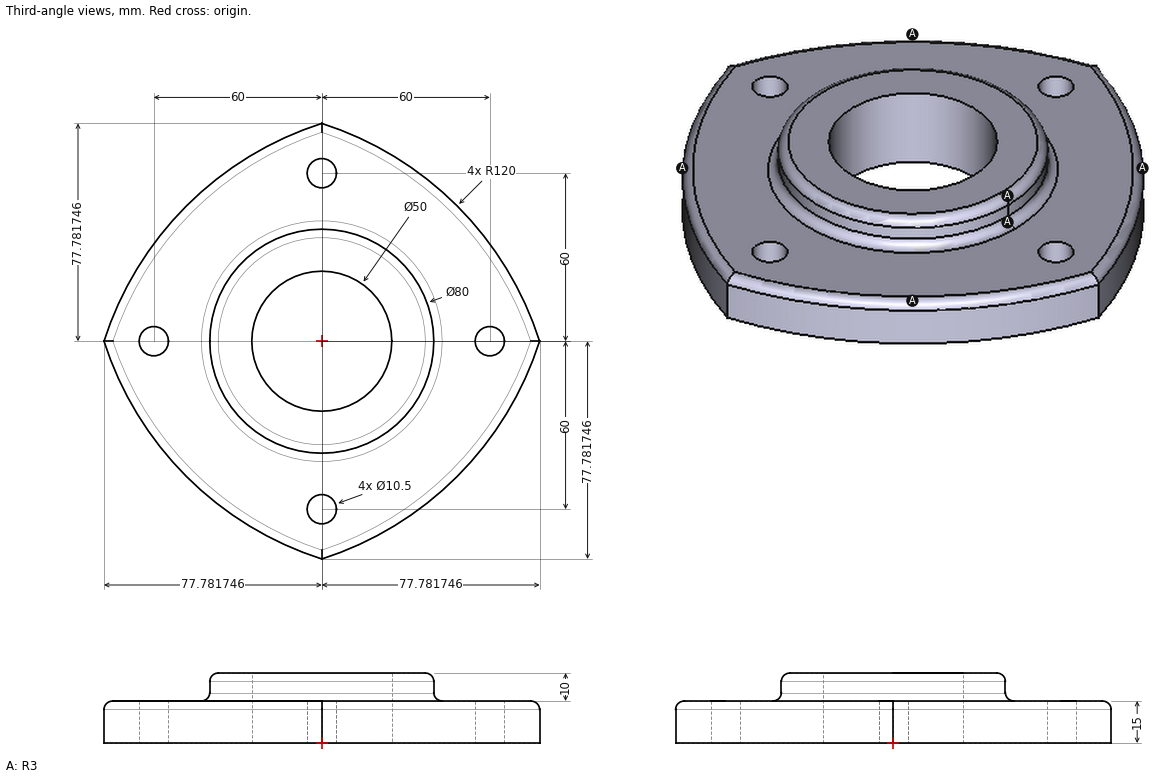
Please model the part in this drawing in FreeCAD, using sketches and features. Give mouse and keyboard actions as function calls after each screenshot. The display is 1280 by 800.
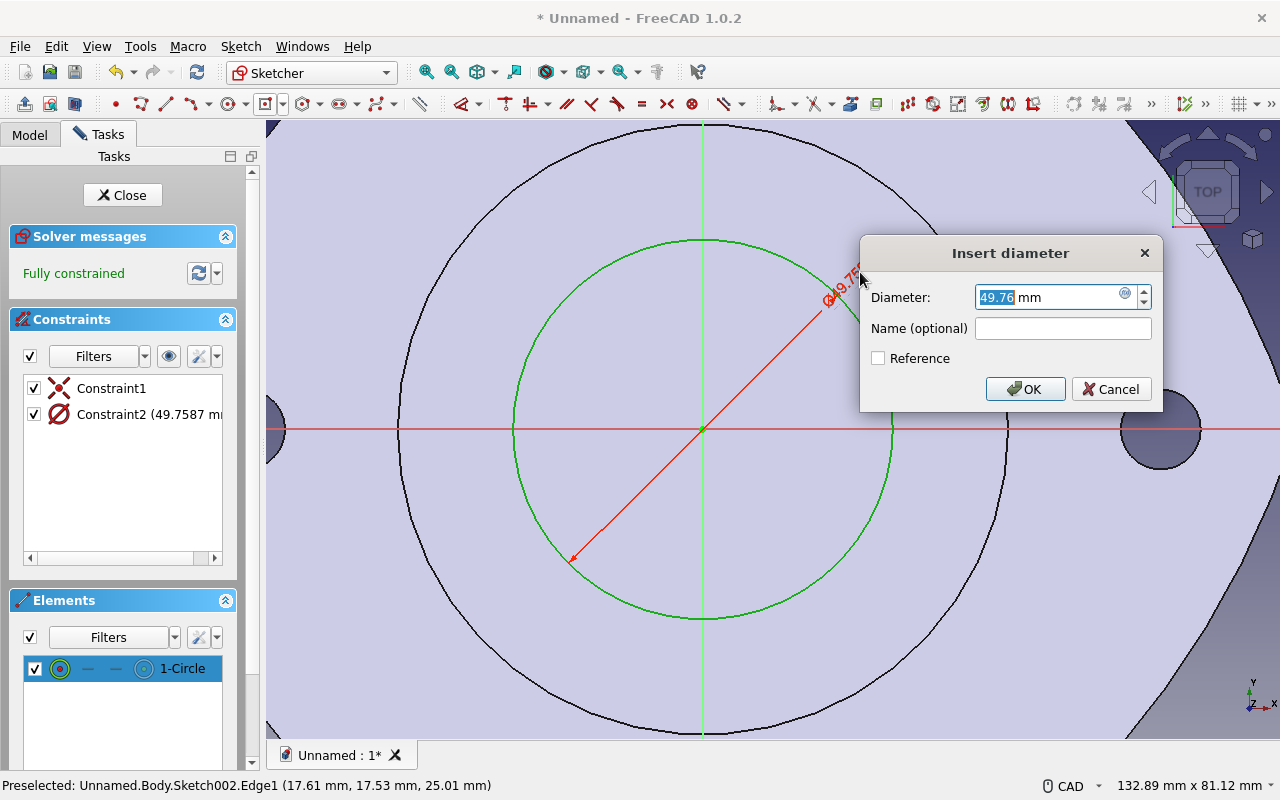
text(50)
key(Return)
key(Escape)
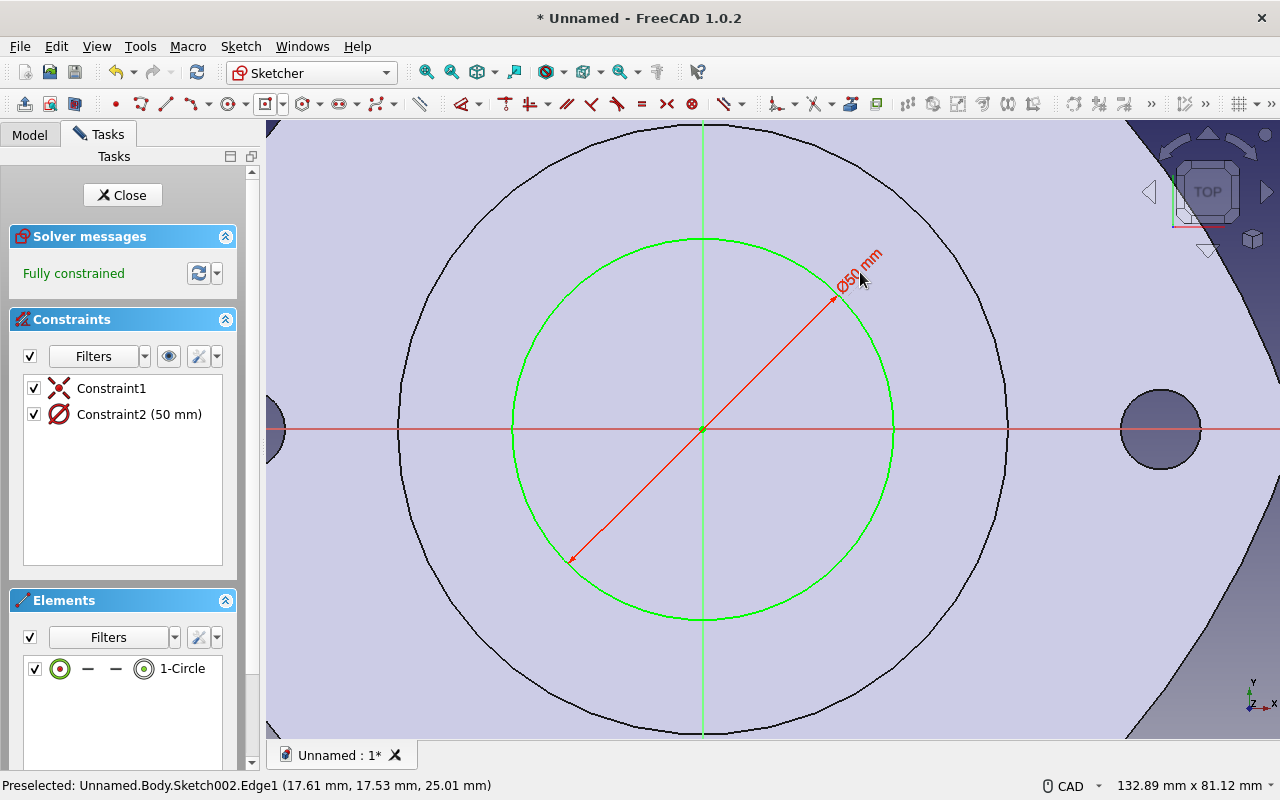
click(123, 195)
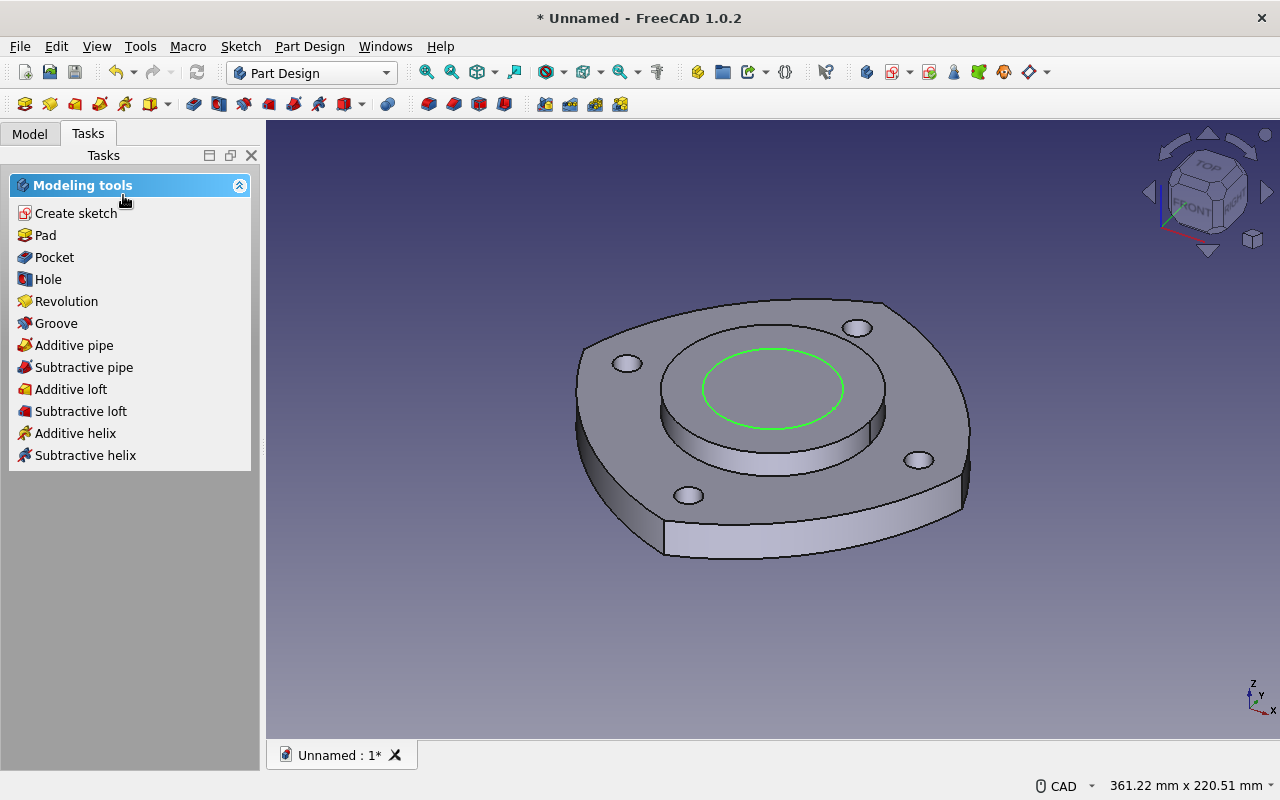
click(194, 104)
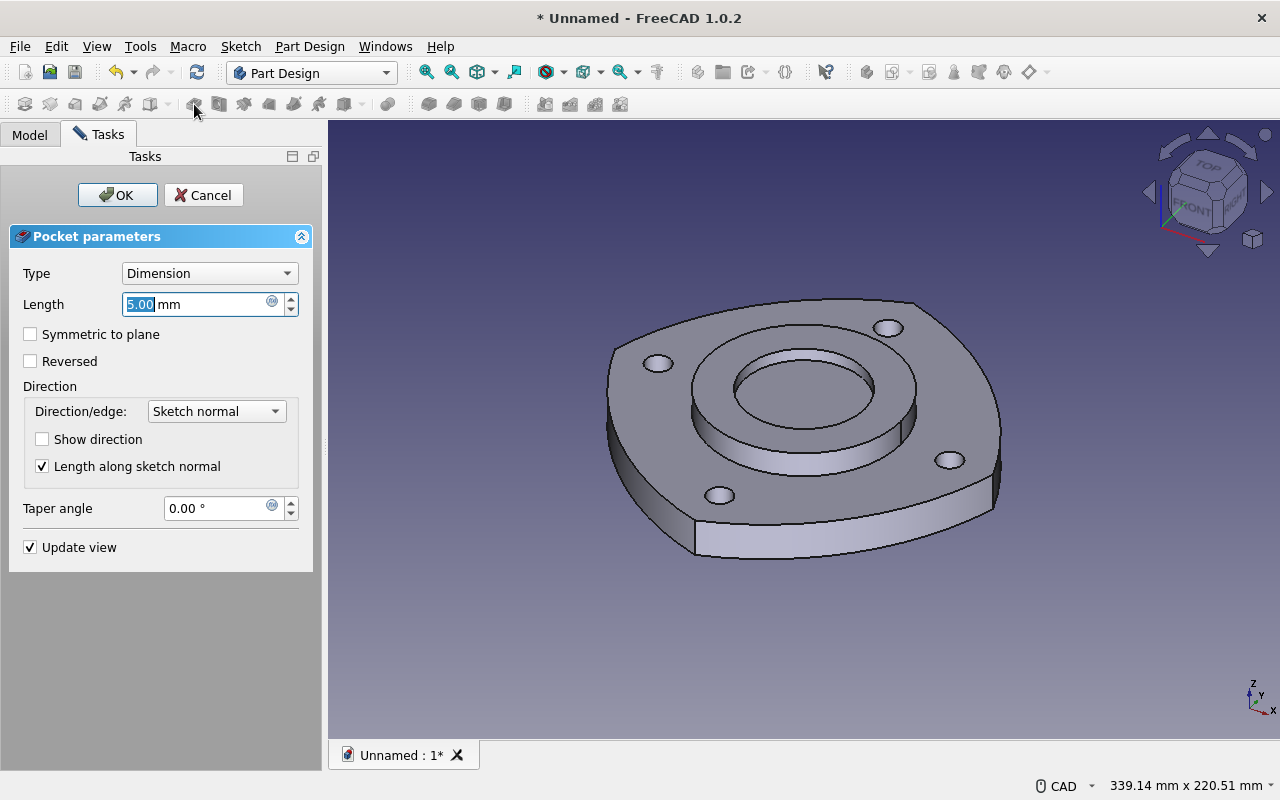
click(210, 274)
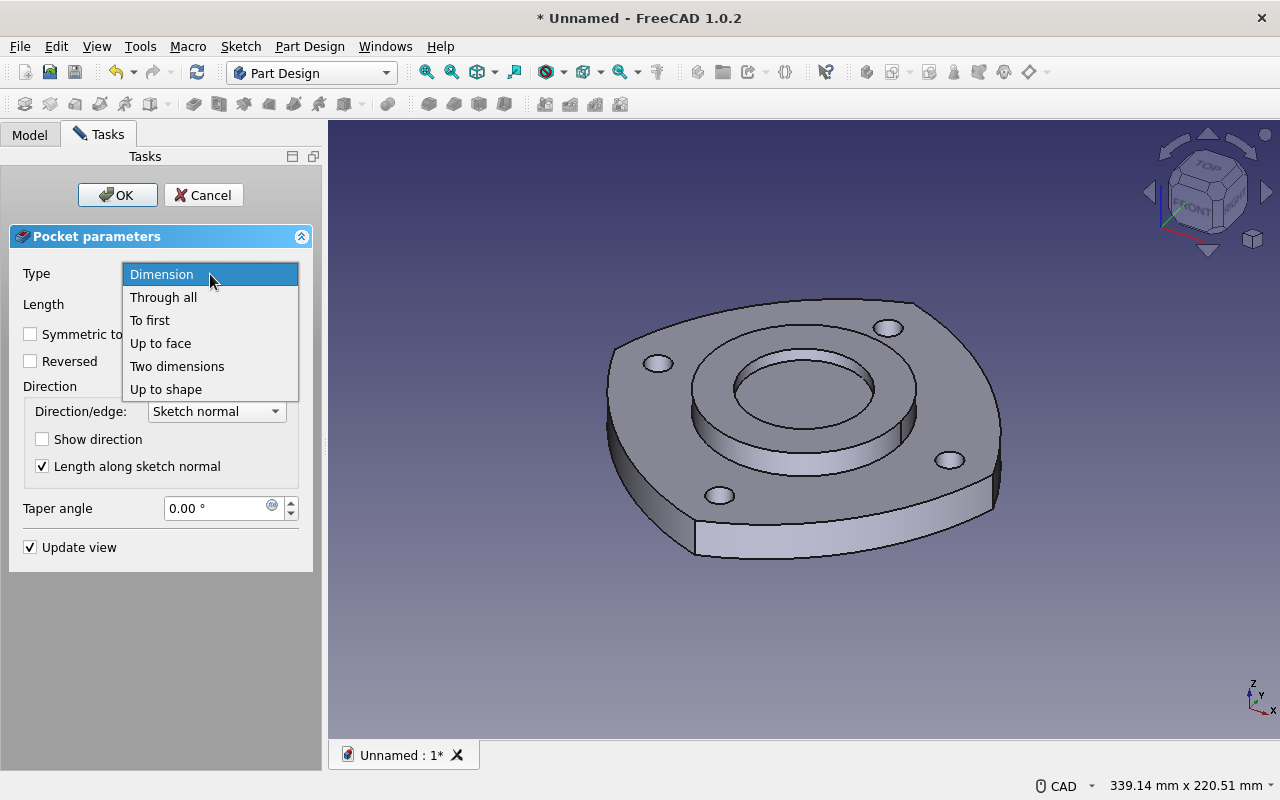
click(208, 298)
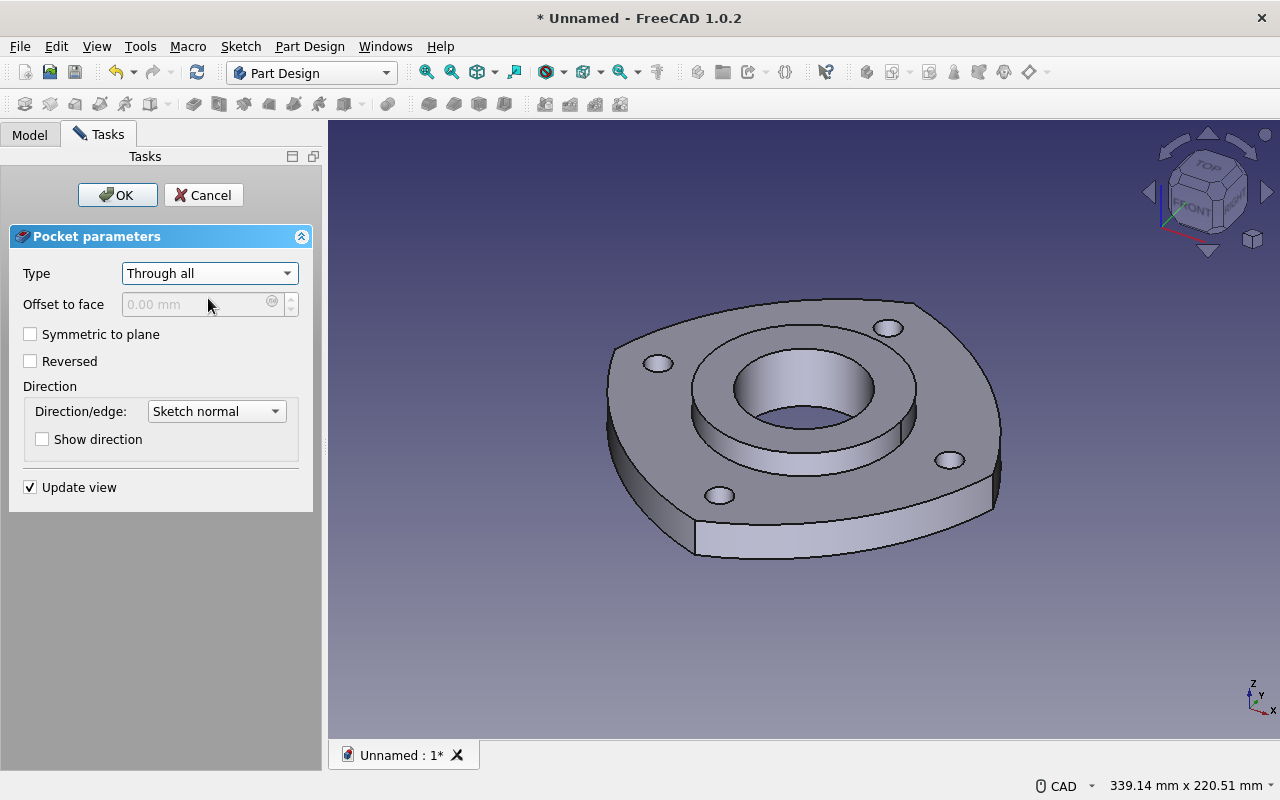
click(118, 195)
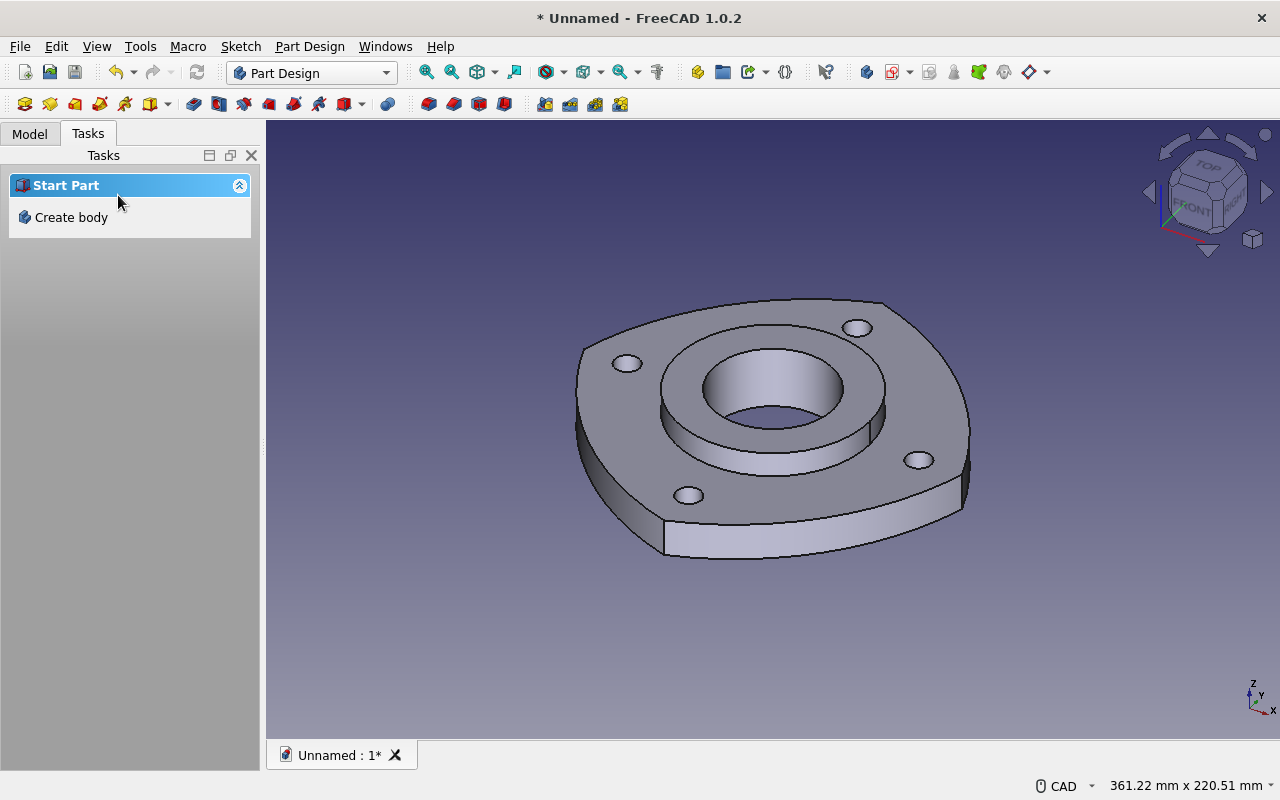
click(823, 517)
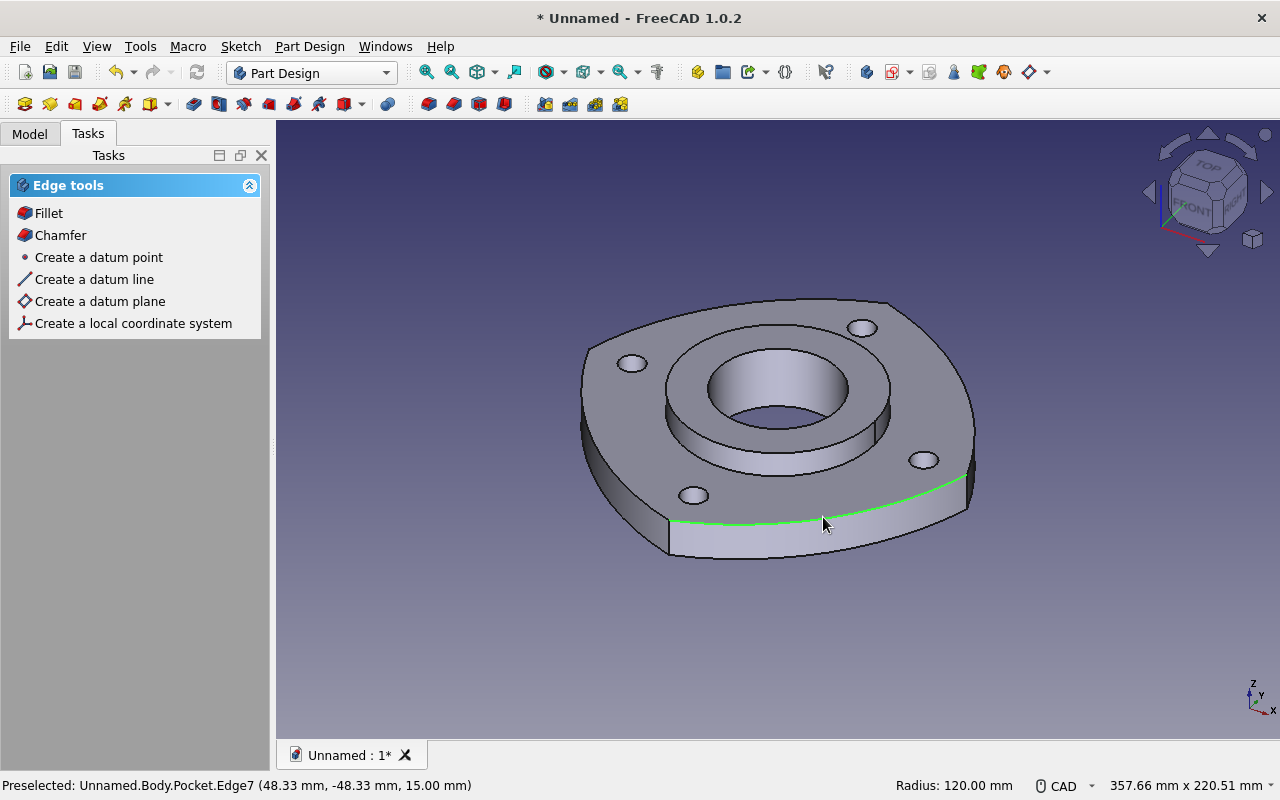
click(954, 365, ctrl)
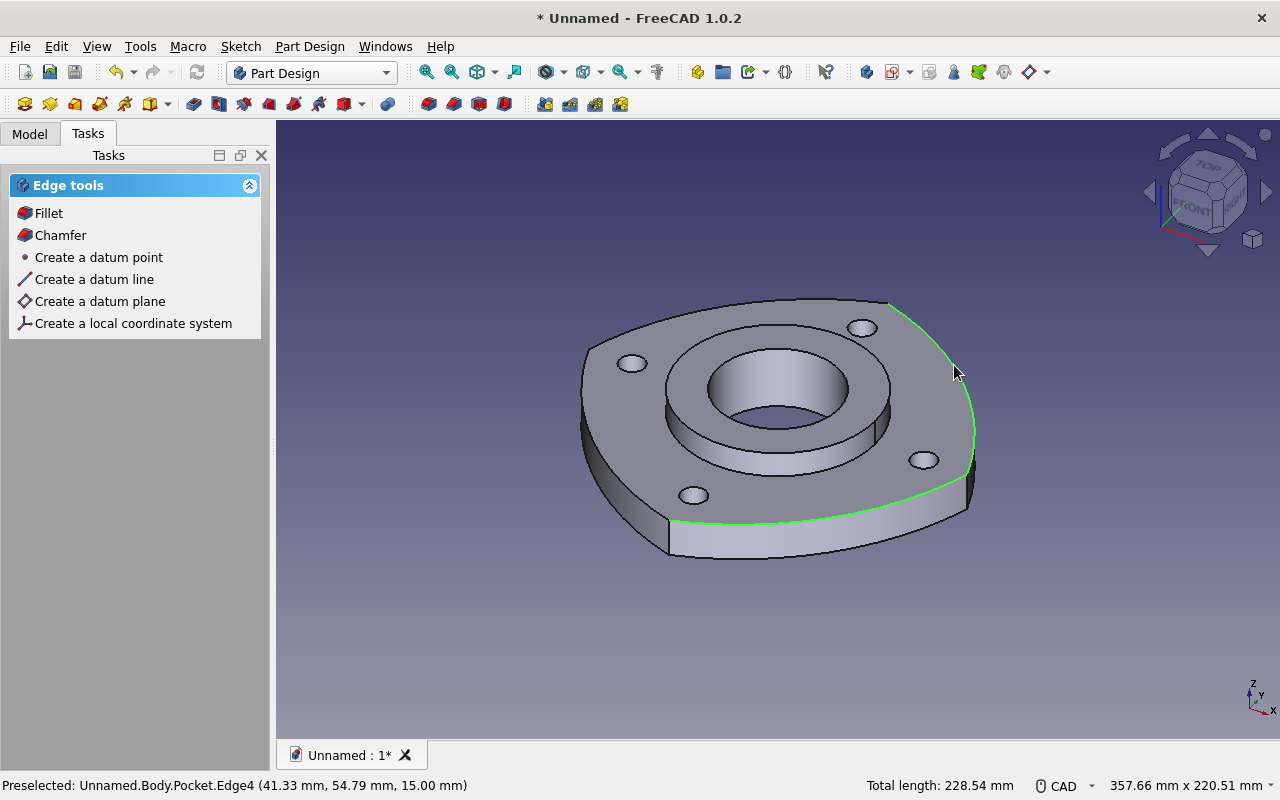
click(666, 395, ctrl)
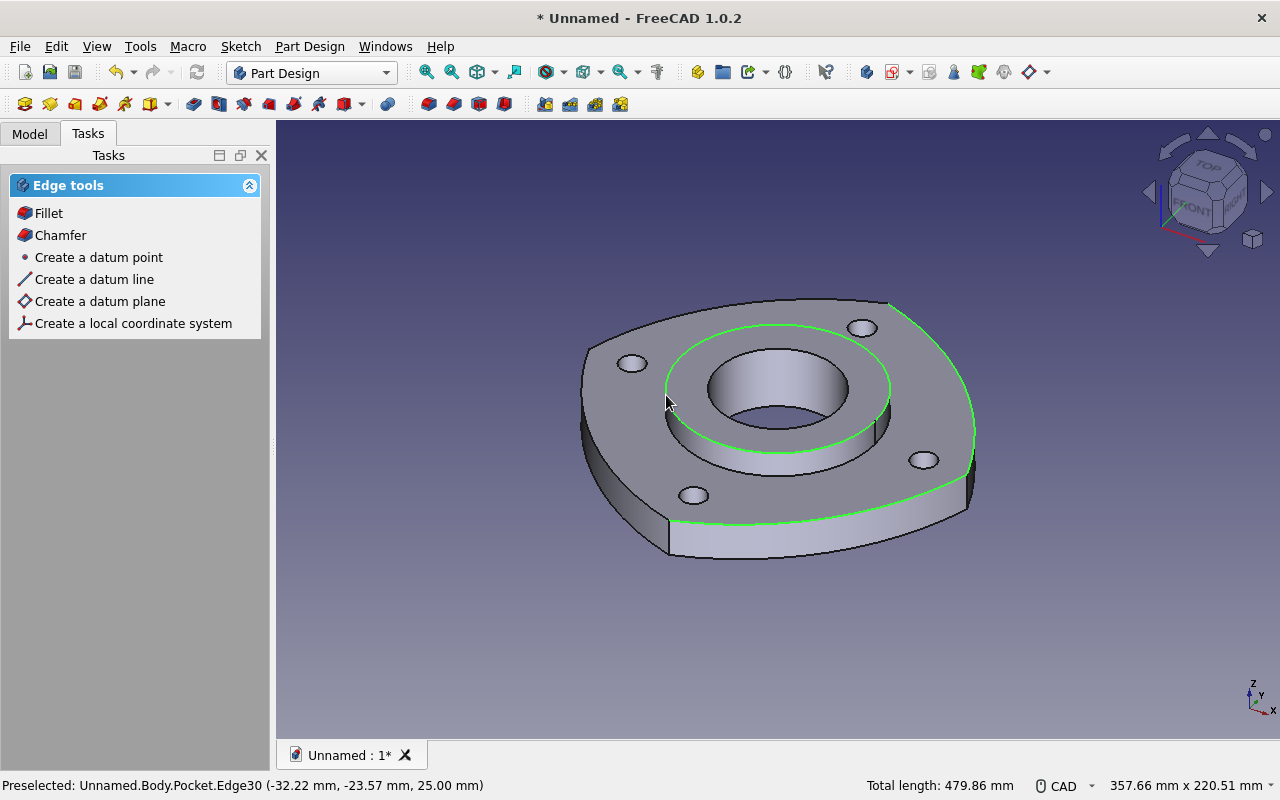
click(593, 439, ctrl)